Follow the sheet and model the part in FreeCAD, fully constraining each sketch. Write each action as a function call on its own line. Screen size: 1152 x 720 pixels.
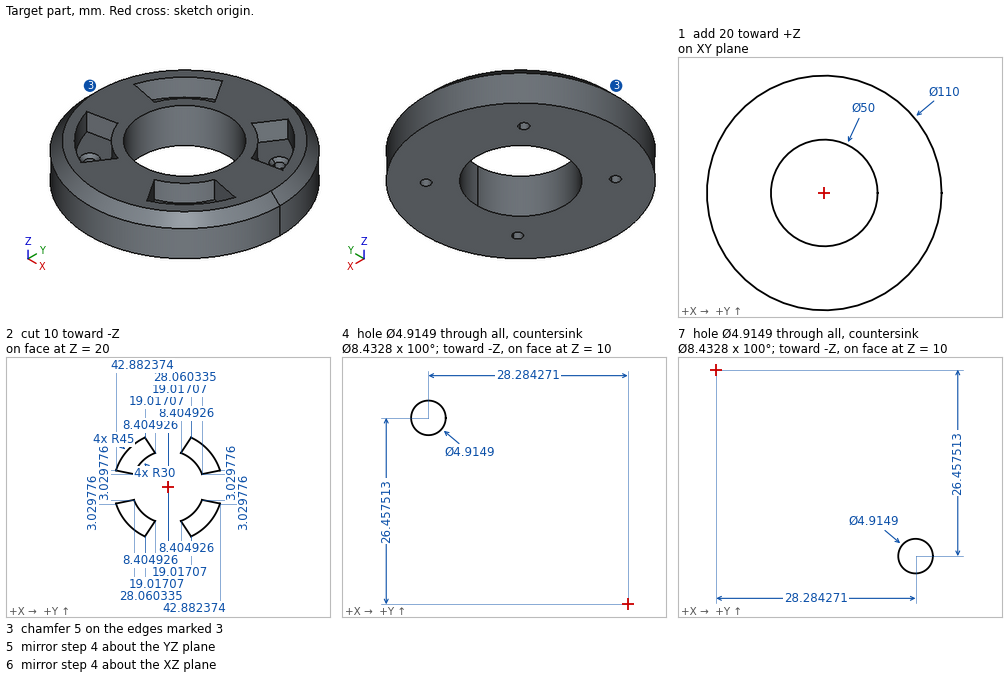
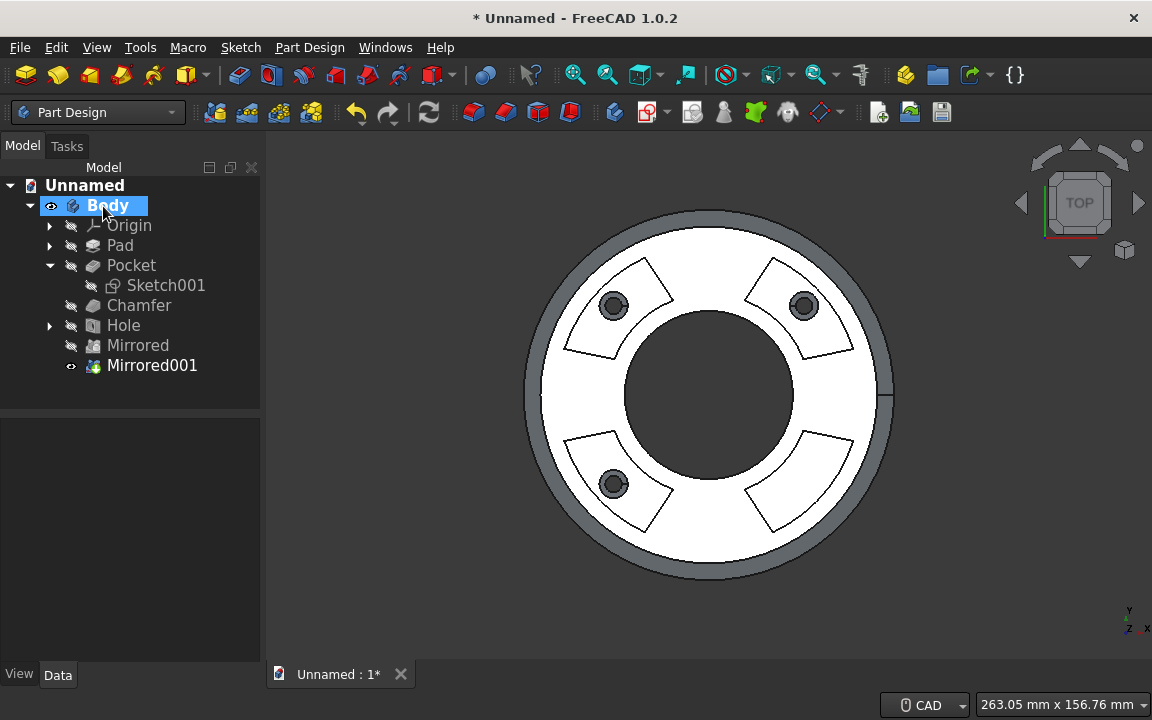
click(783, 495)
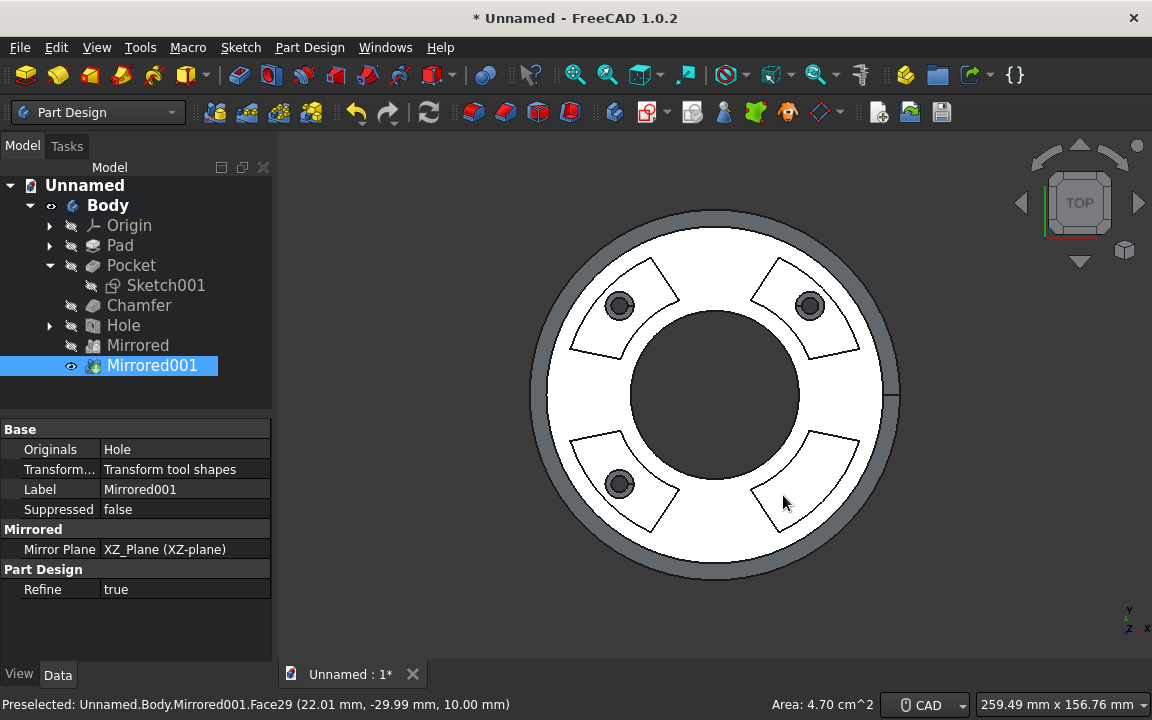
click(648, 112)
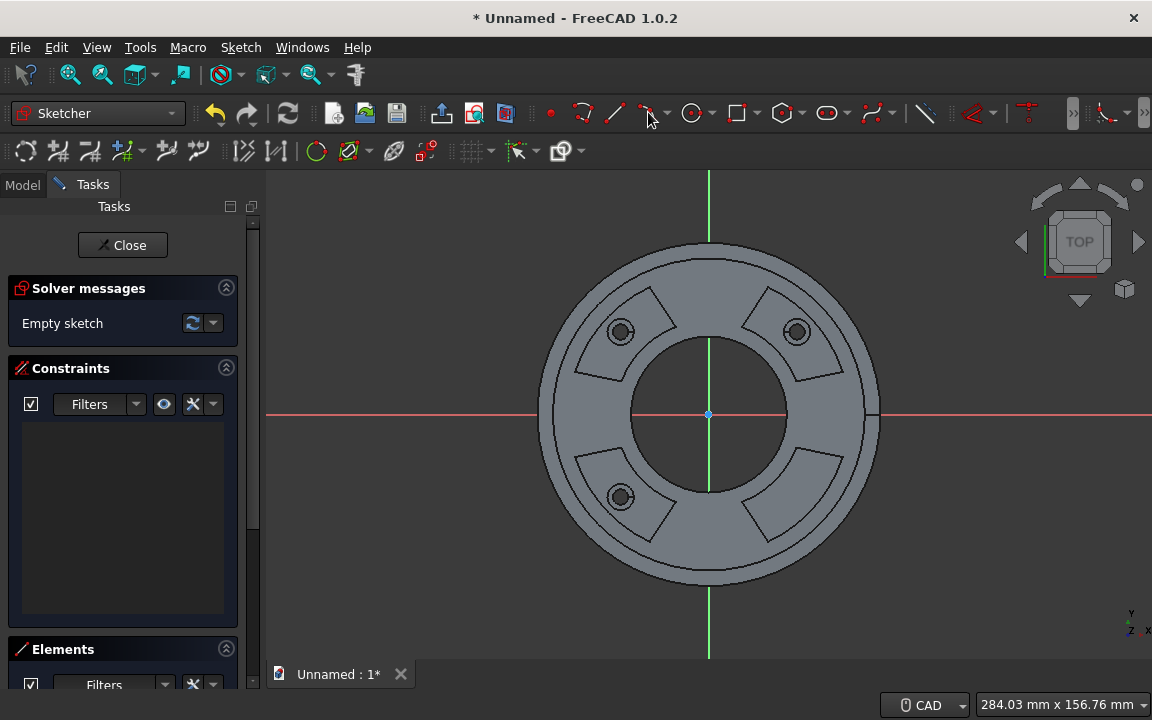
scroll(805, 501, up, 15)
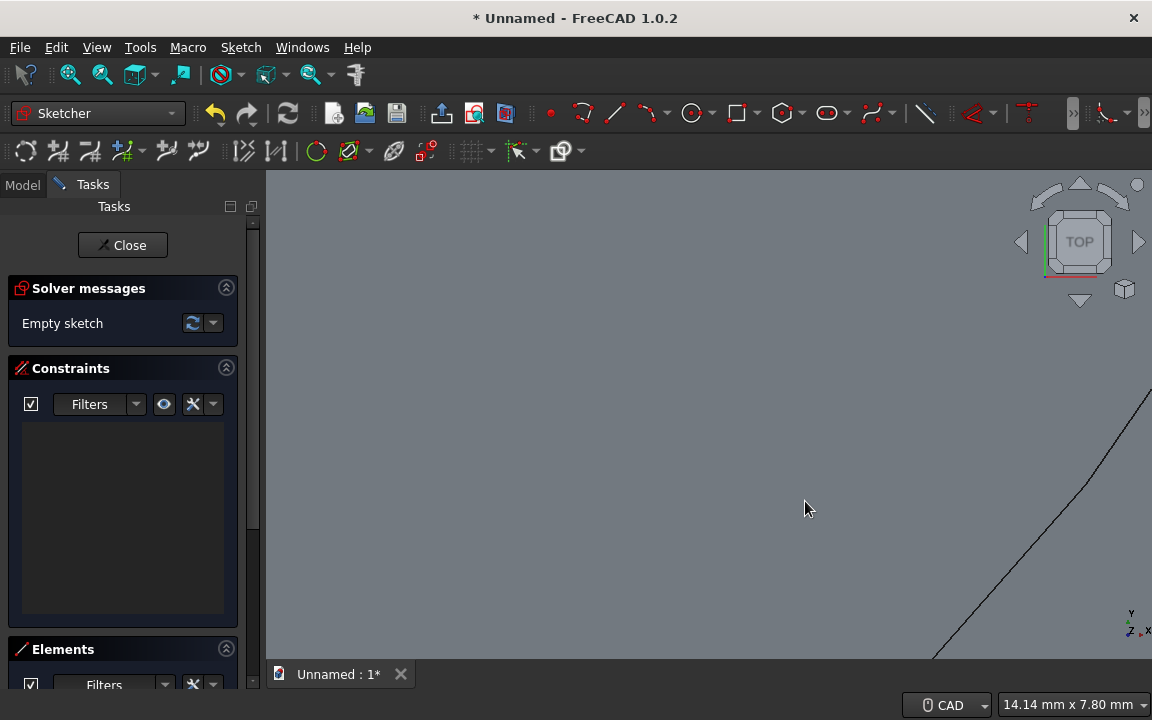
click(692, 114)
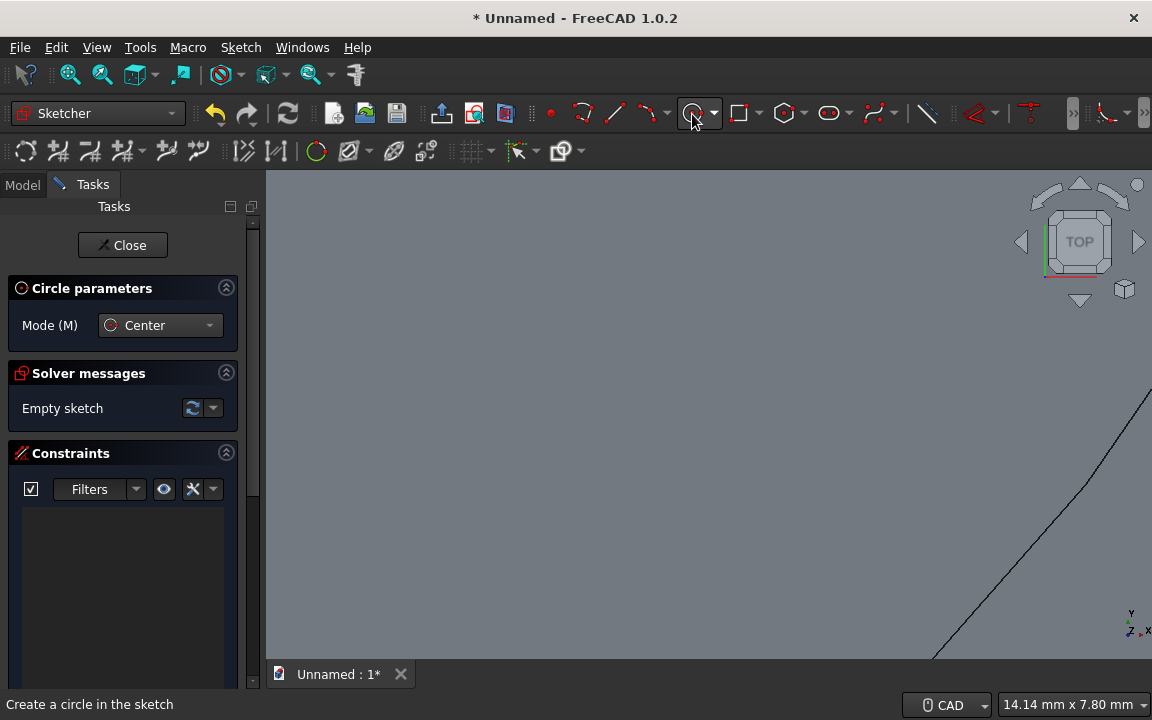
click(635, 408)
click(744, 299)
key(Escape)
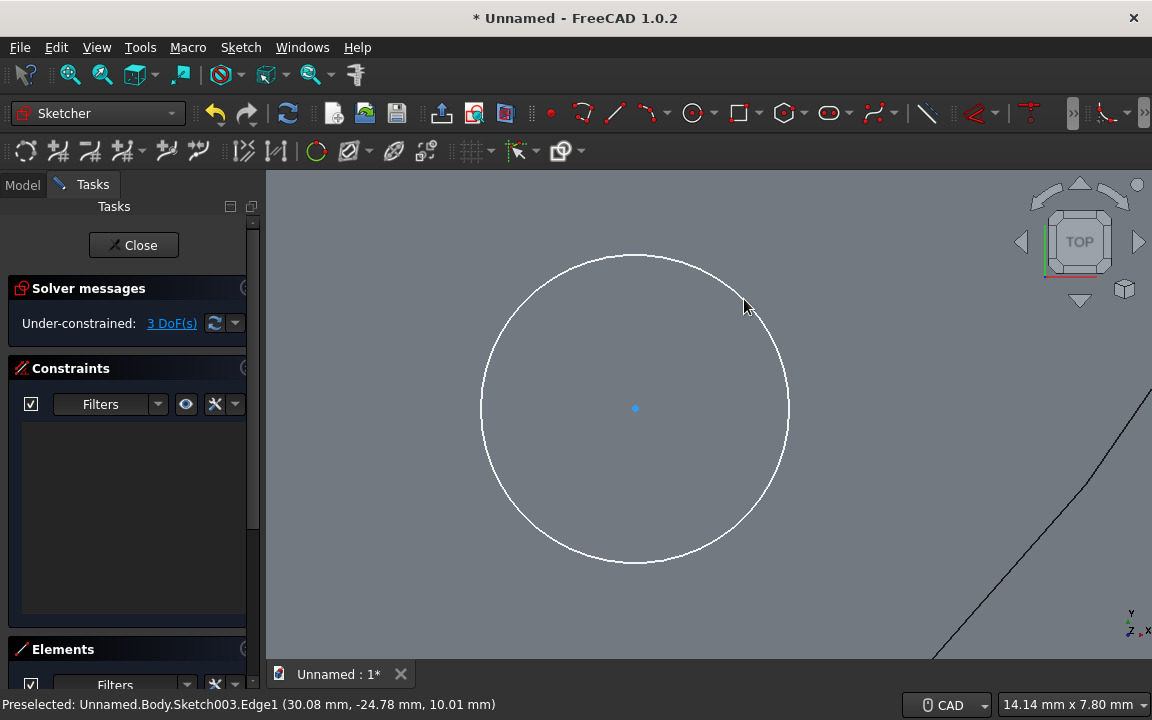
click(974, 114)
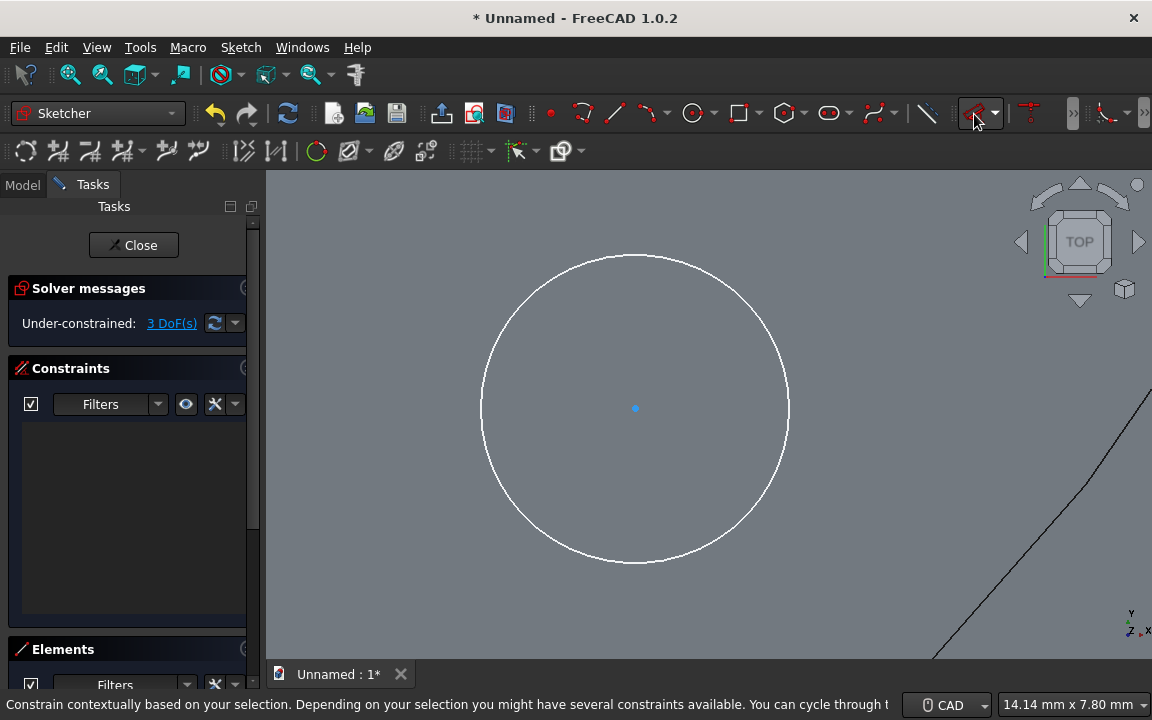
click(744, 300)
click(767, 277)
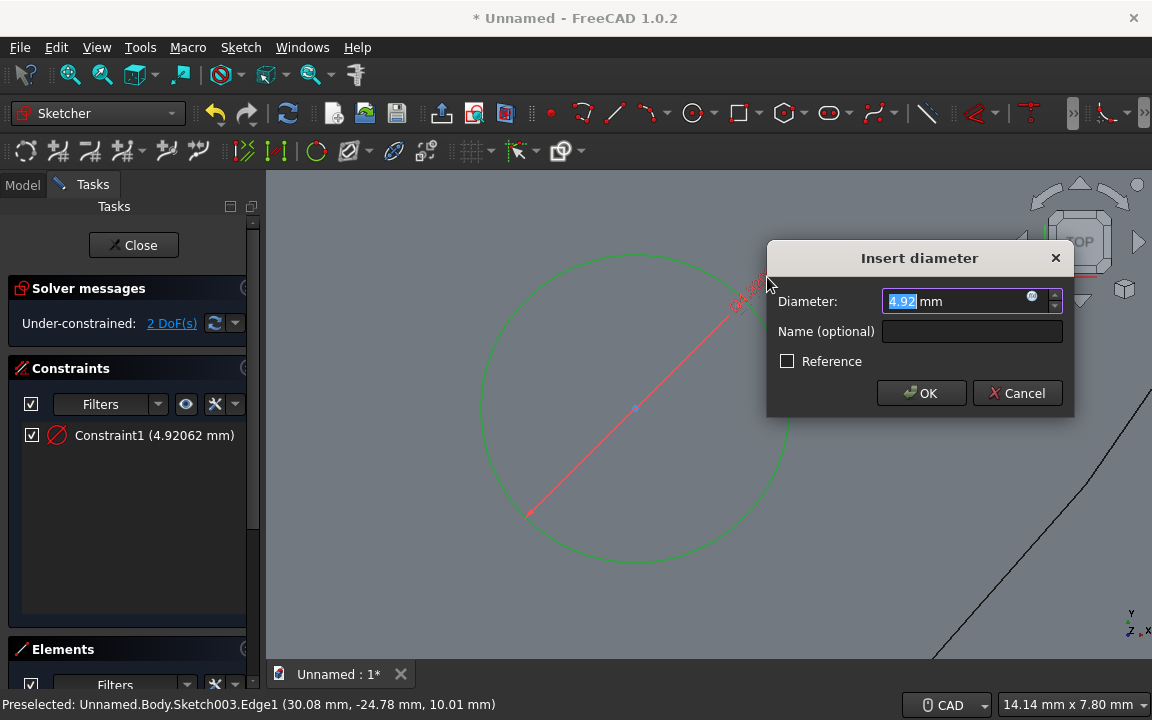
text(4.9149)
key(Return)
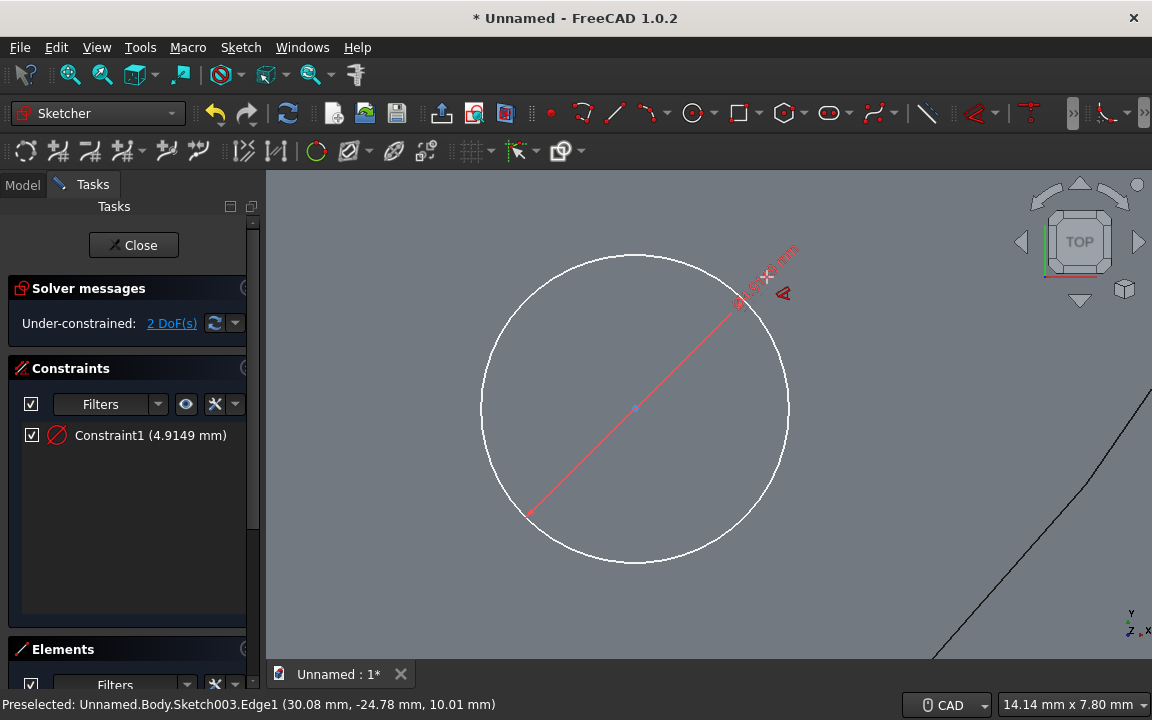
click(635, 409)
click(464, 443)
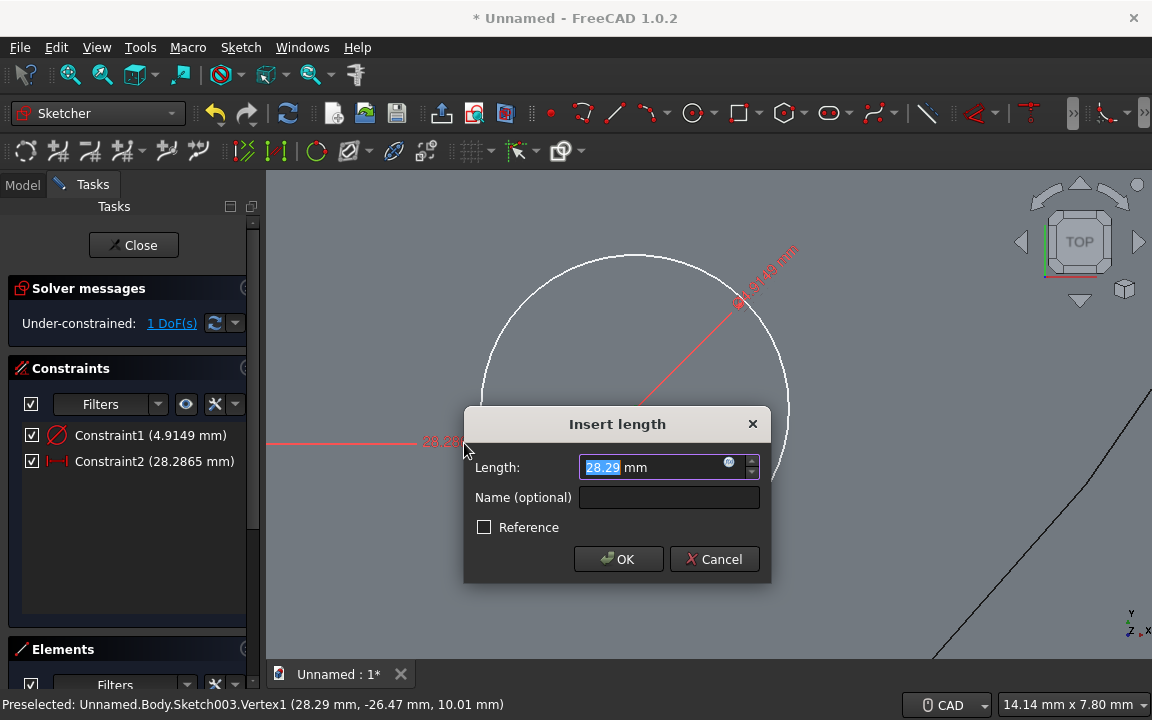
text(28.284271)
key(Return)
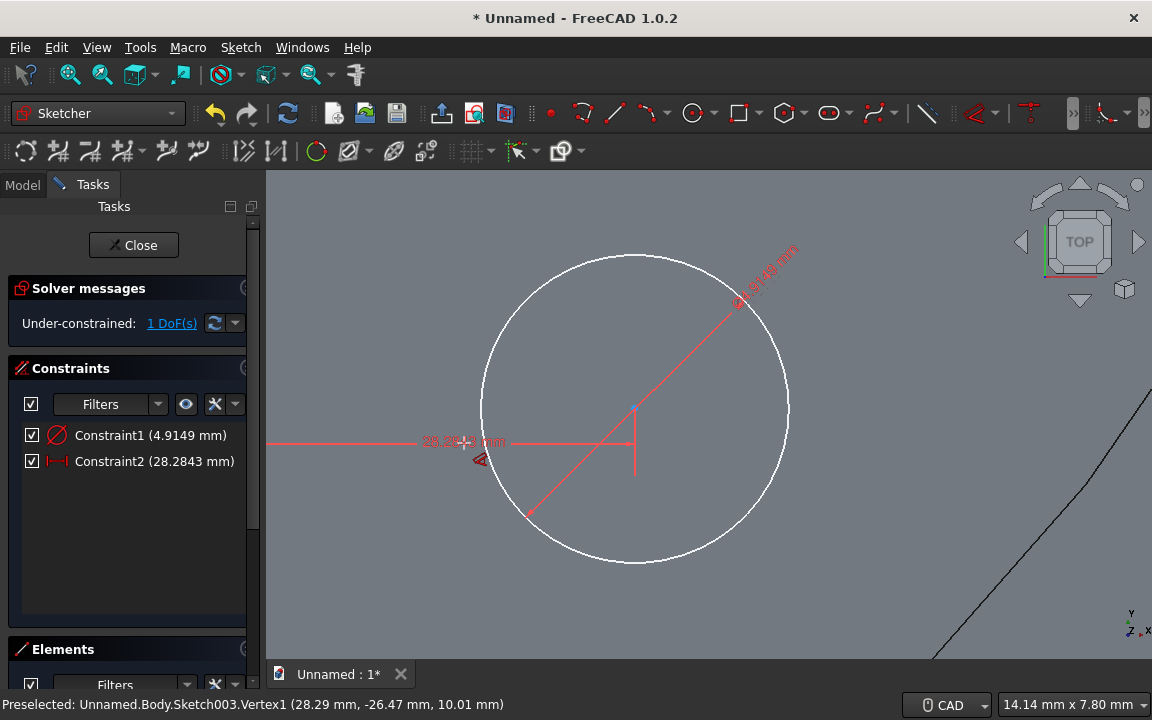
click(635, 409)
click(669, 303)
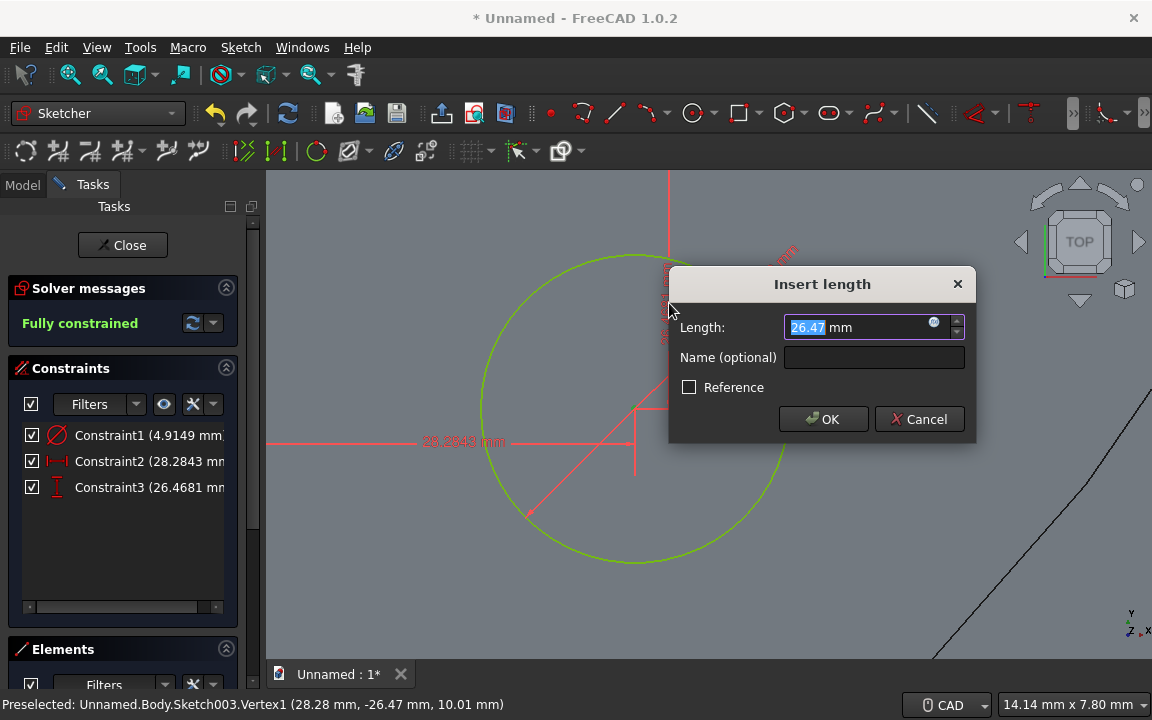
text(26.457513)
key(Return)
key(Escape)